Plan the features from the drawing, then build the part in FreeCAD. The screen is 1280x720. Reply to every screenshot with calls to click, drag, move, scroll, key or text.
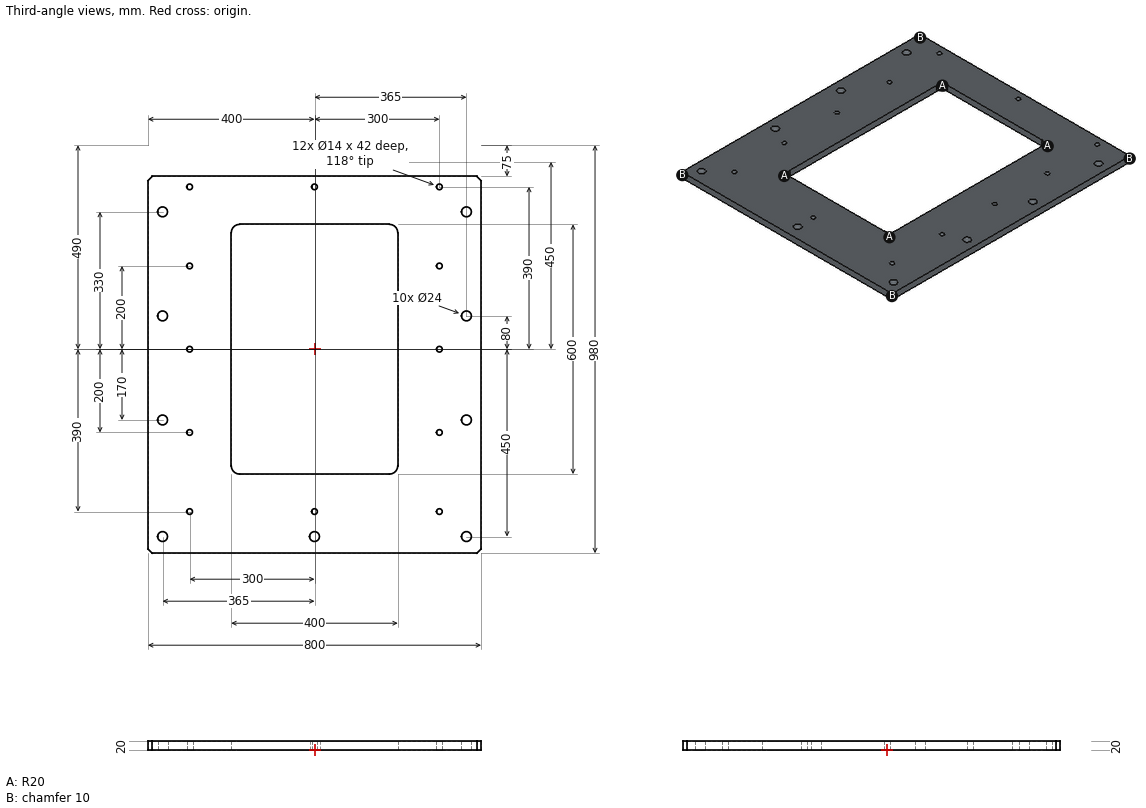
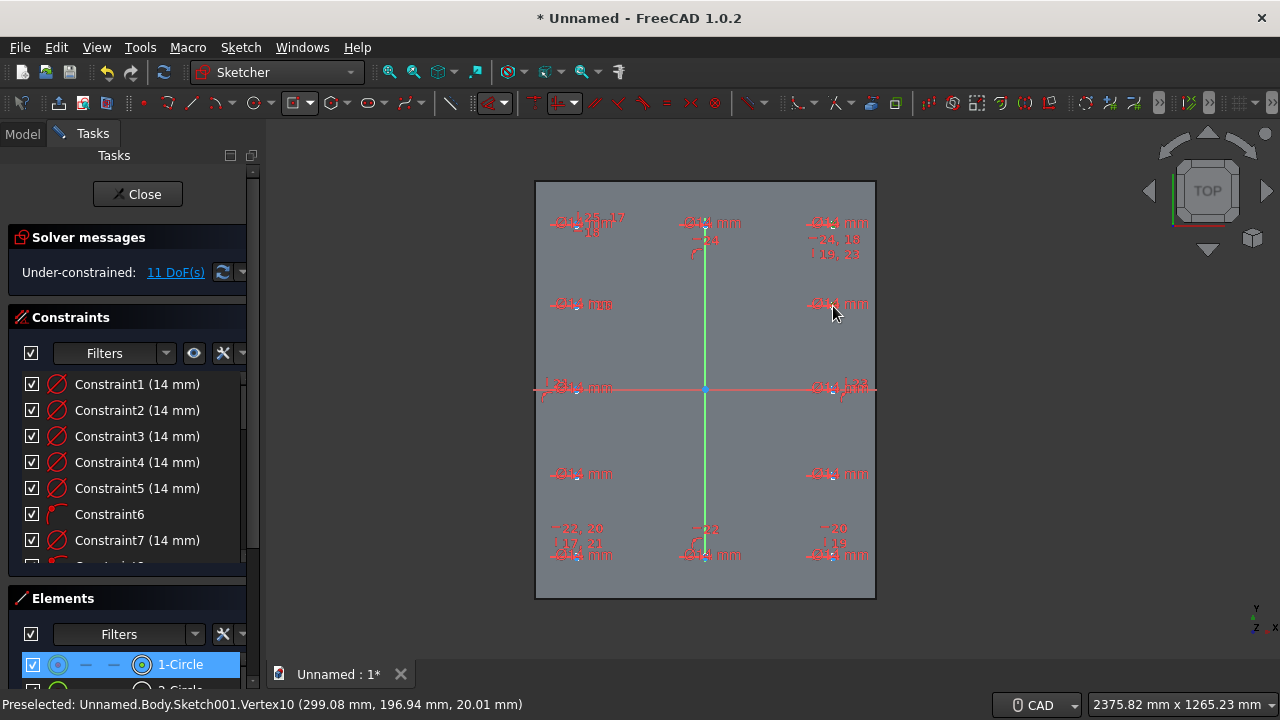
key(v)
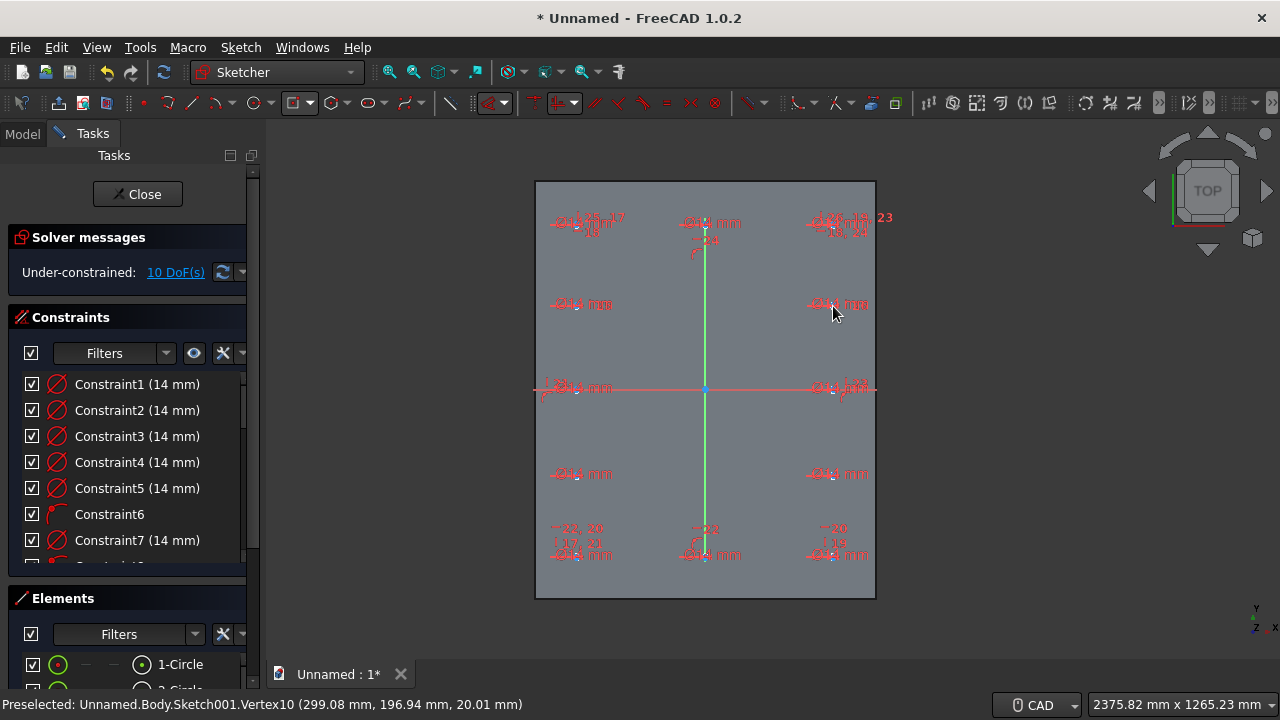
click(577, 306)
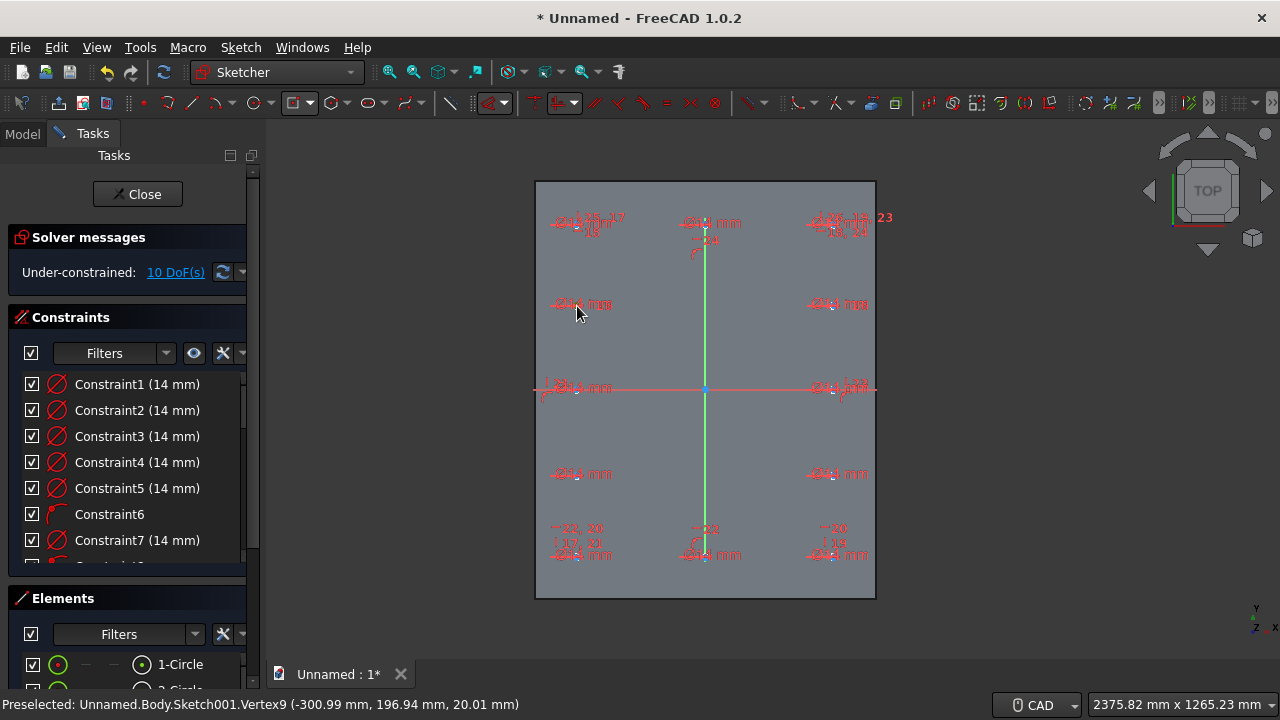
click(833, 306)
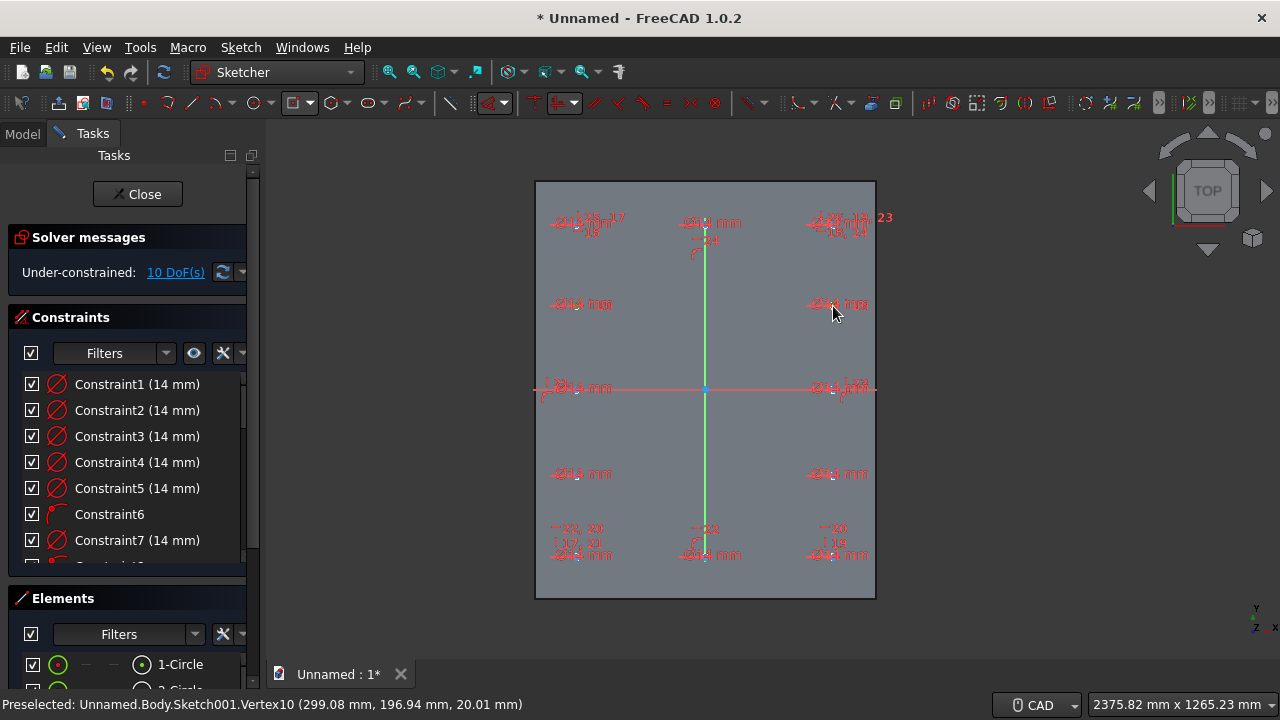
click(576, 104)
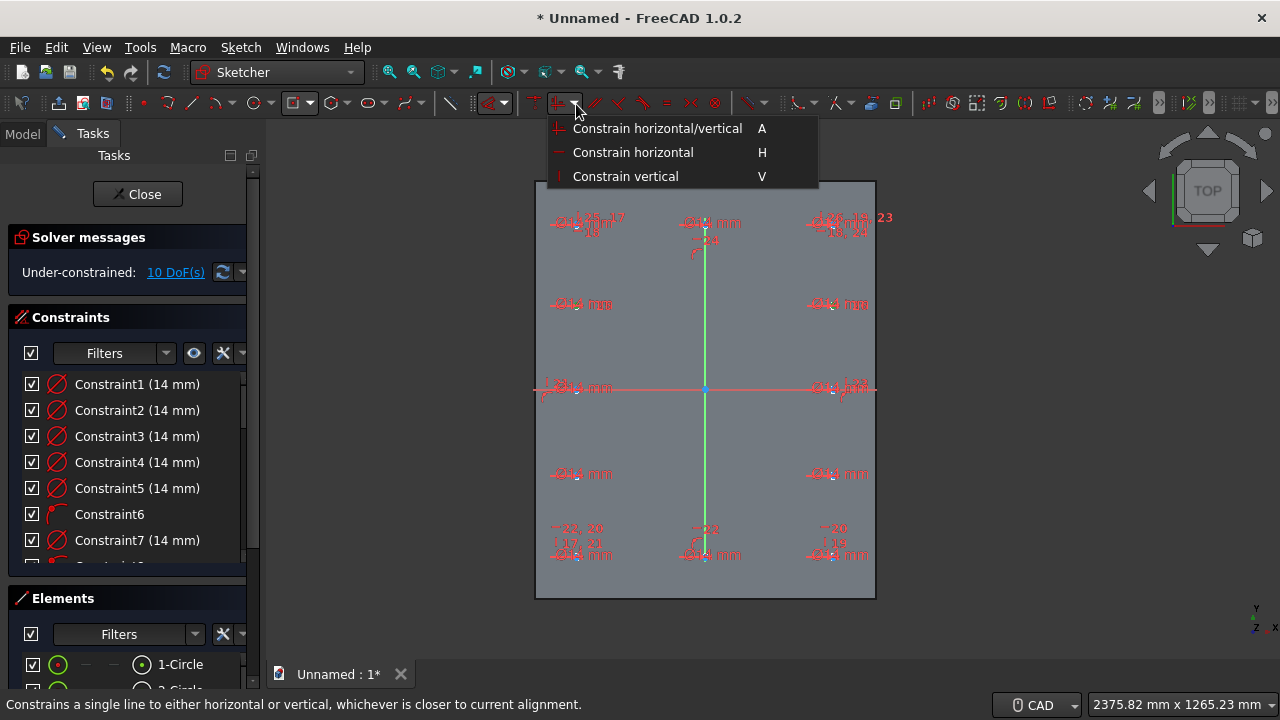
click(683, 152)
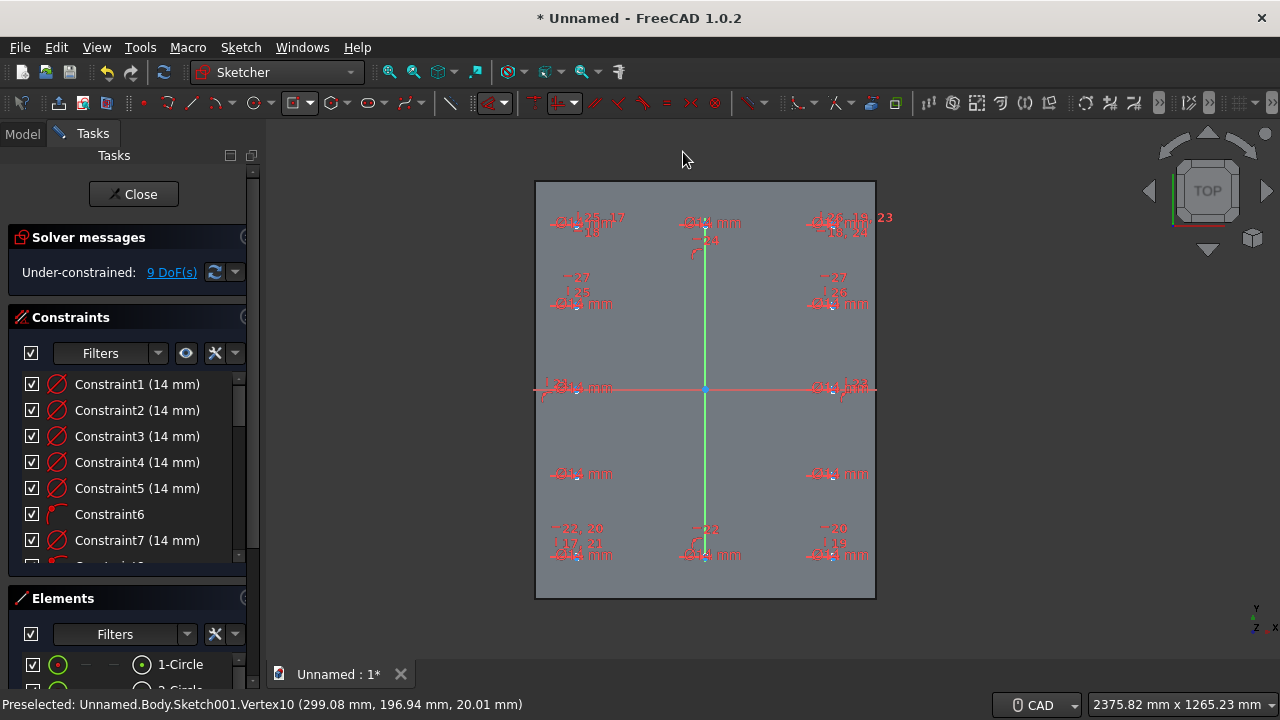
click(577, 557)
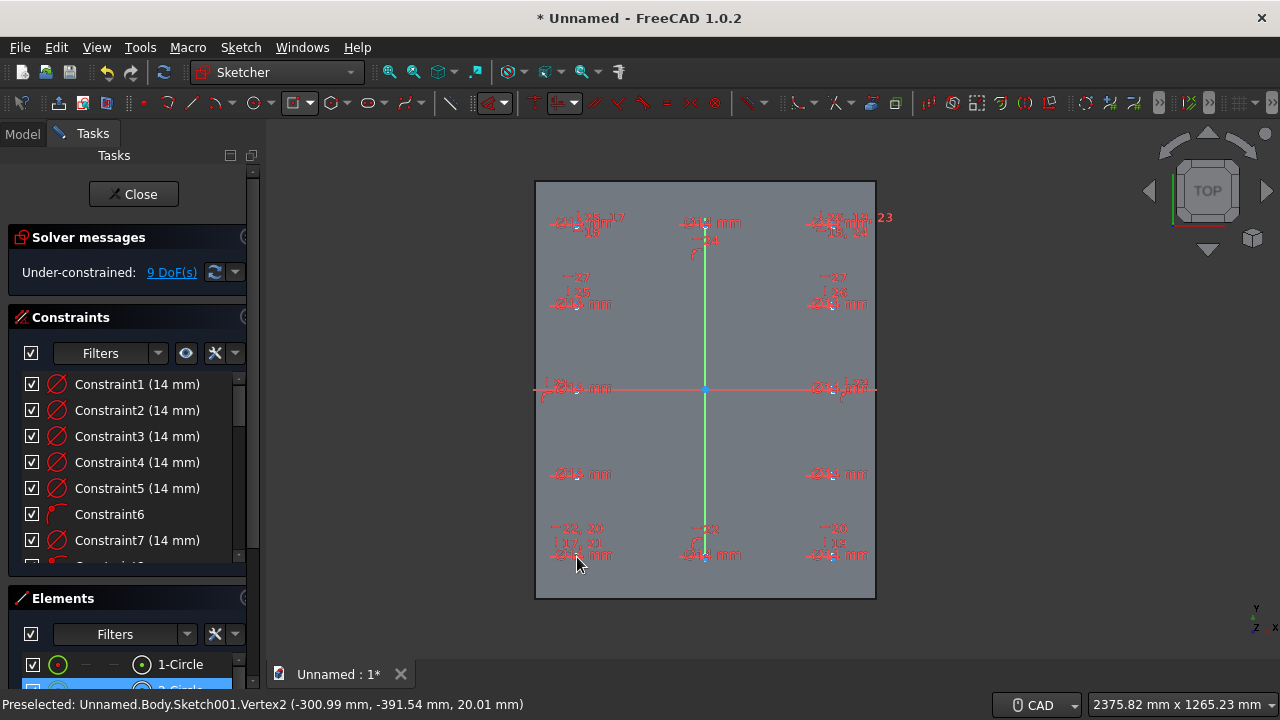
click(577, 476)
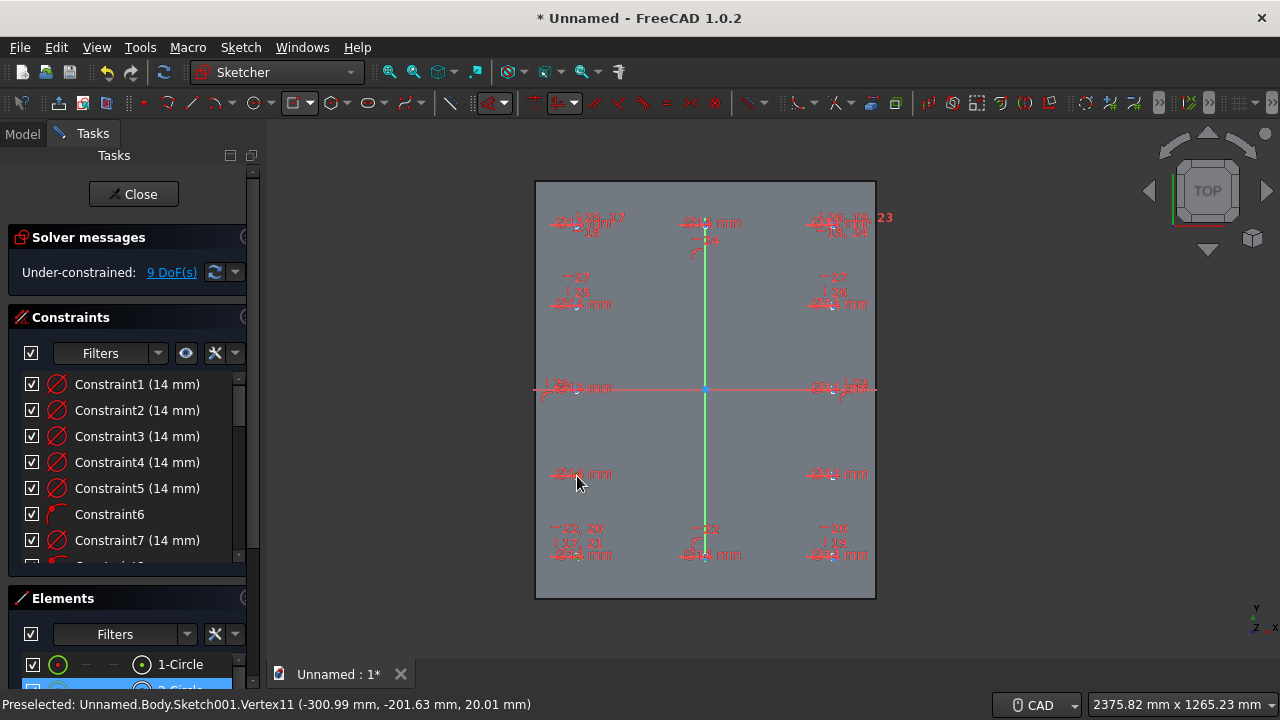
key(v)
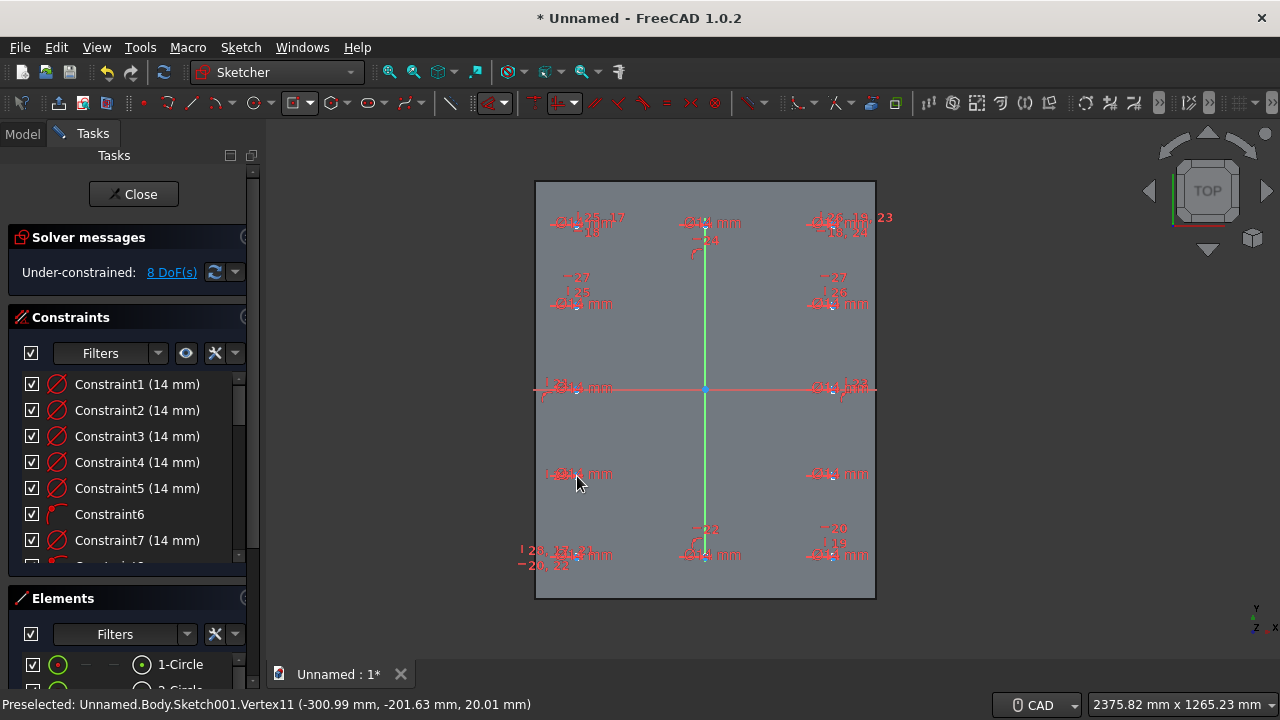
click(833, 557)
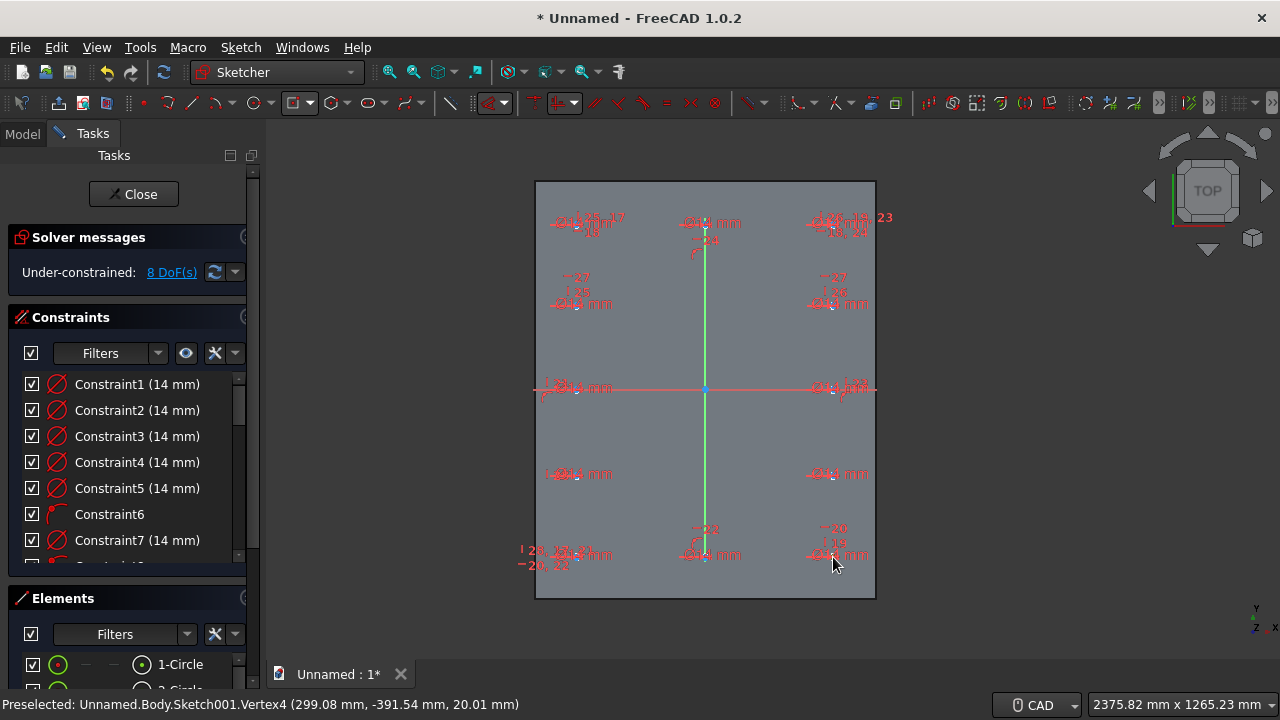
click(833, 476)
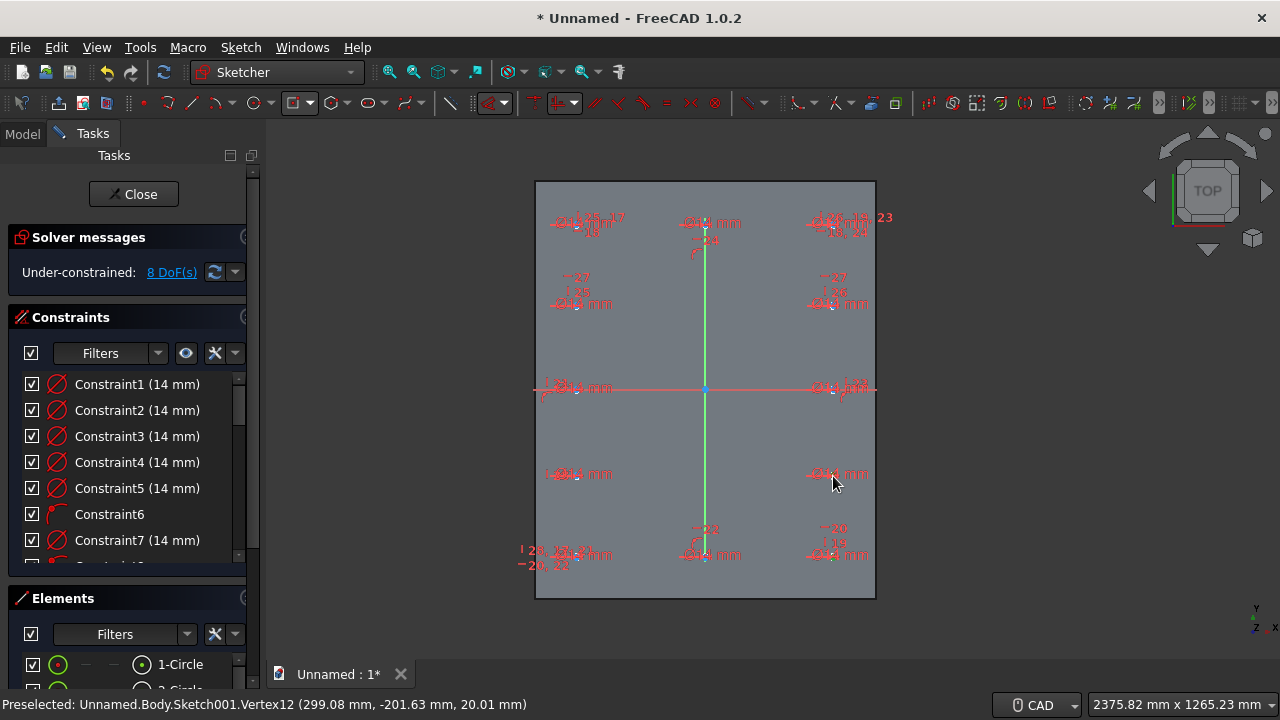
key(v)